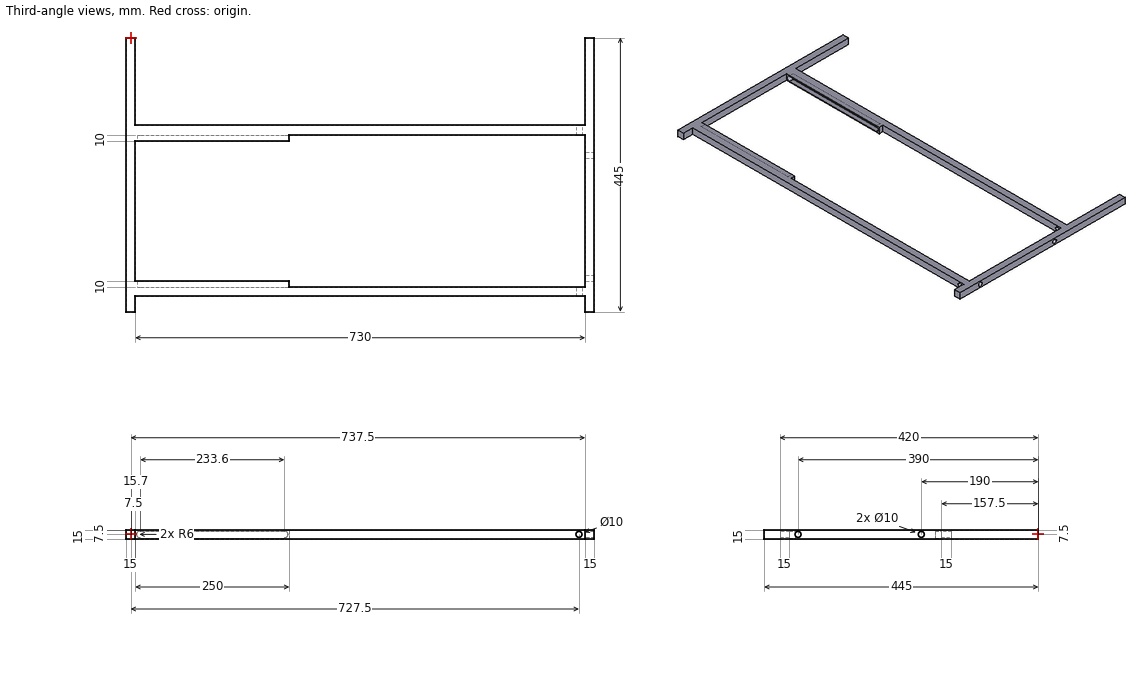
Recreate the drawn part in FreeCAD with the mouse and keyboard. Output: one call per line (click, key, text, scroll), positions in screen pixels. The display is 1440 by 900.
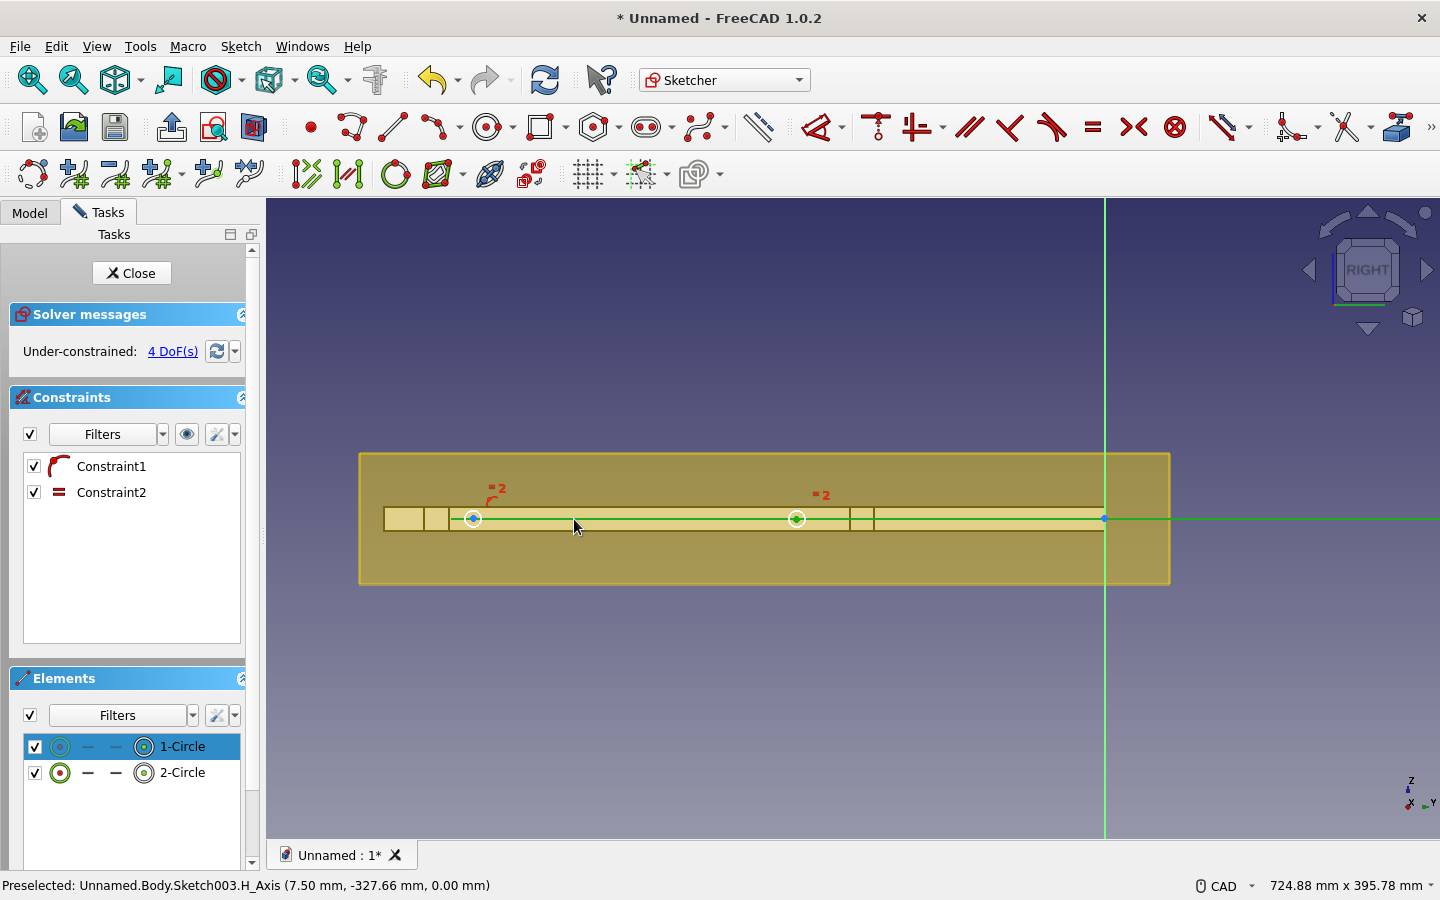
click(876, 128)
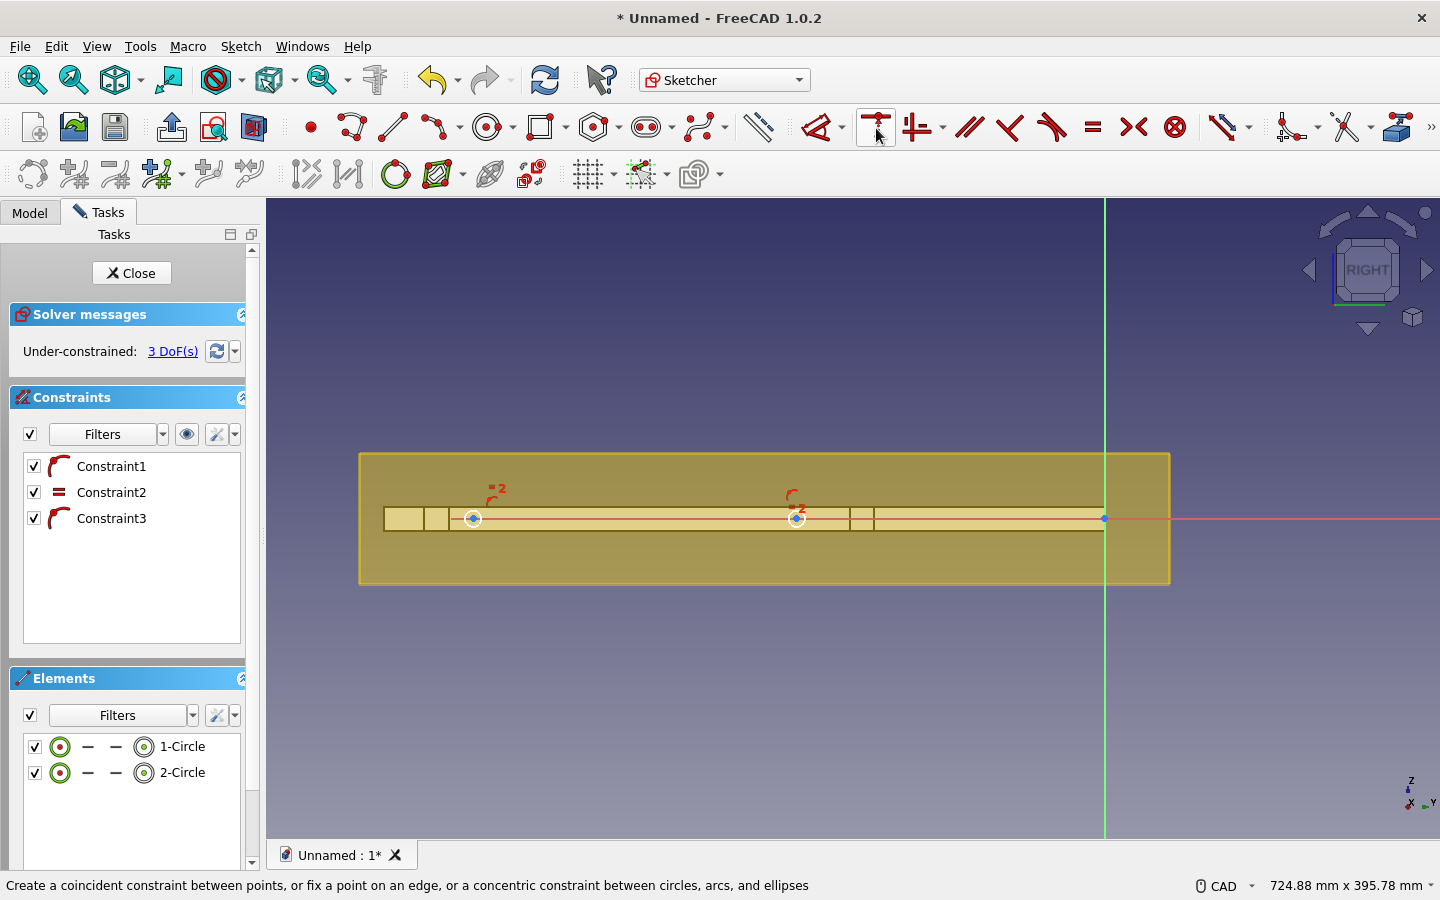
click(816, 128)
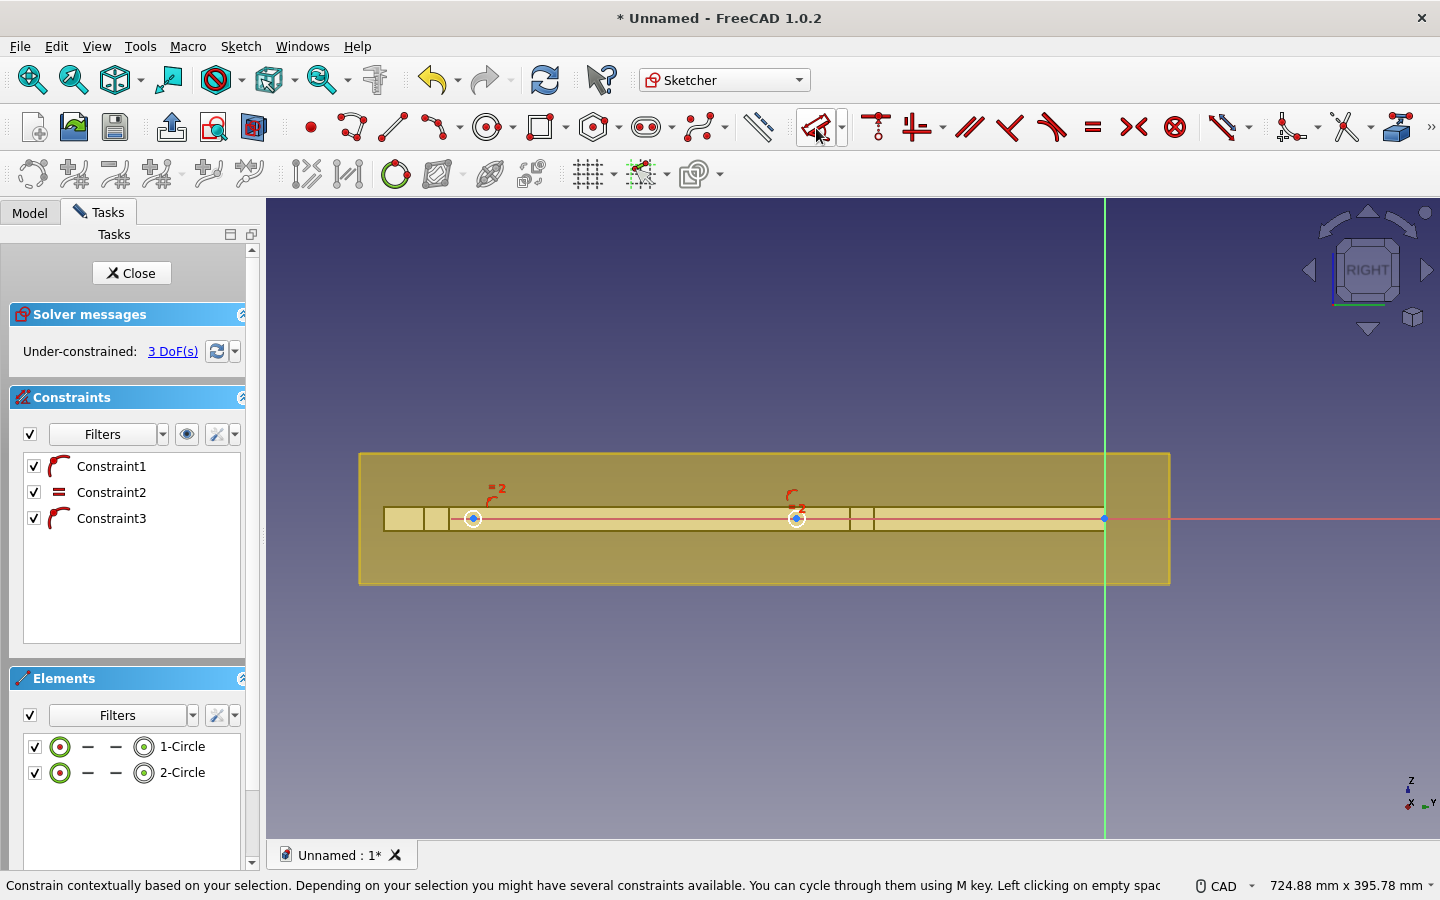
scroll(789, 519, up, 5)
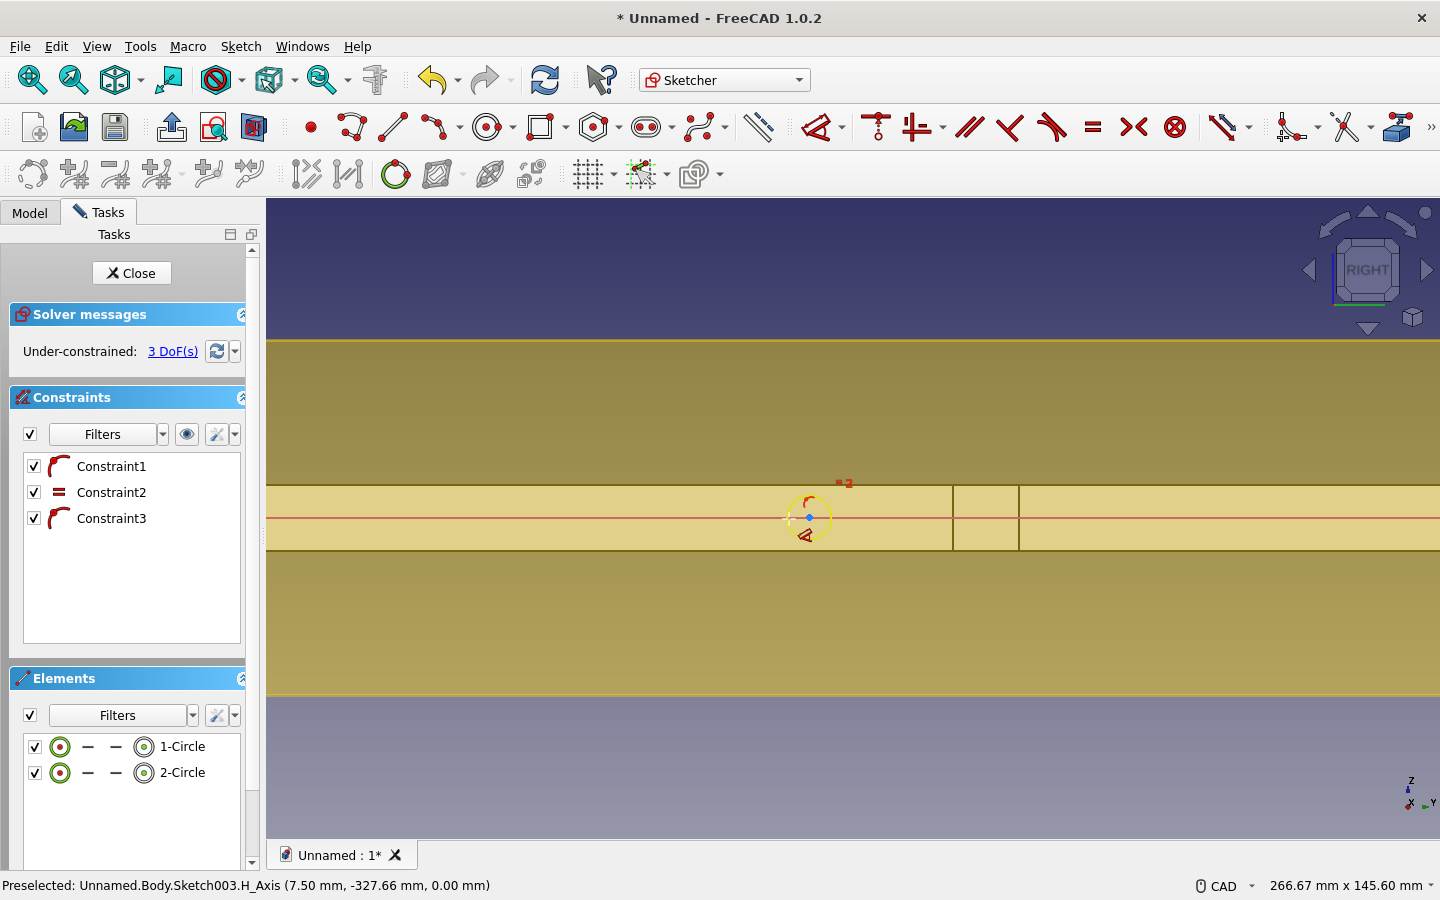
click(787, 517)
click(762, 490)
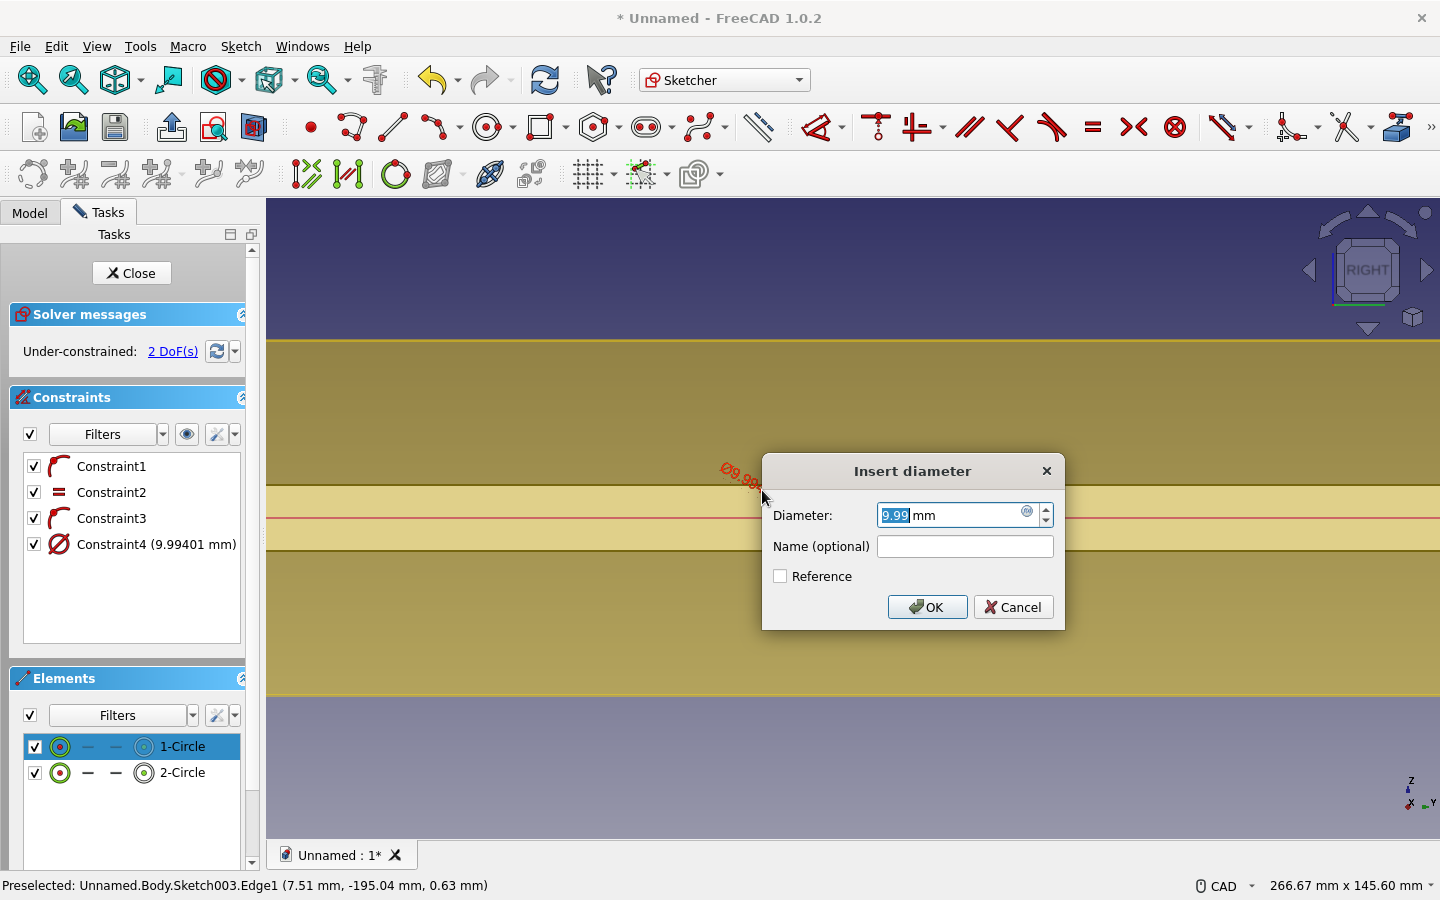
text(10)
key(Return)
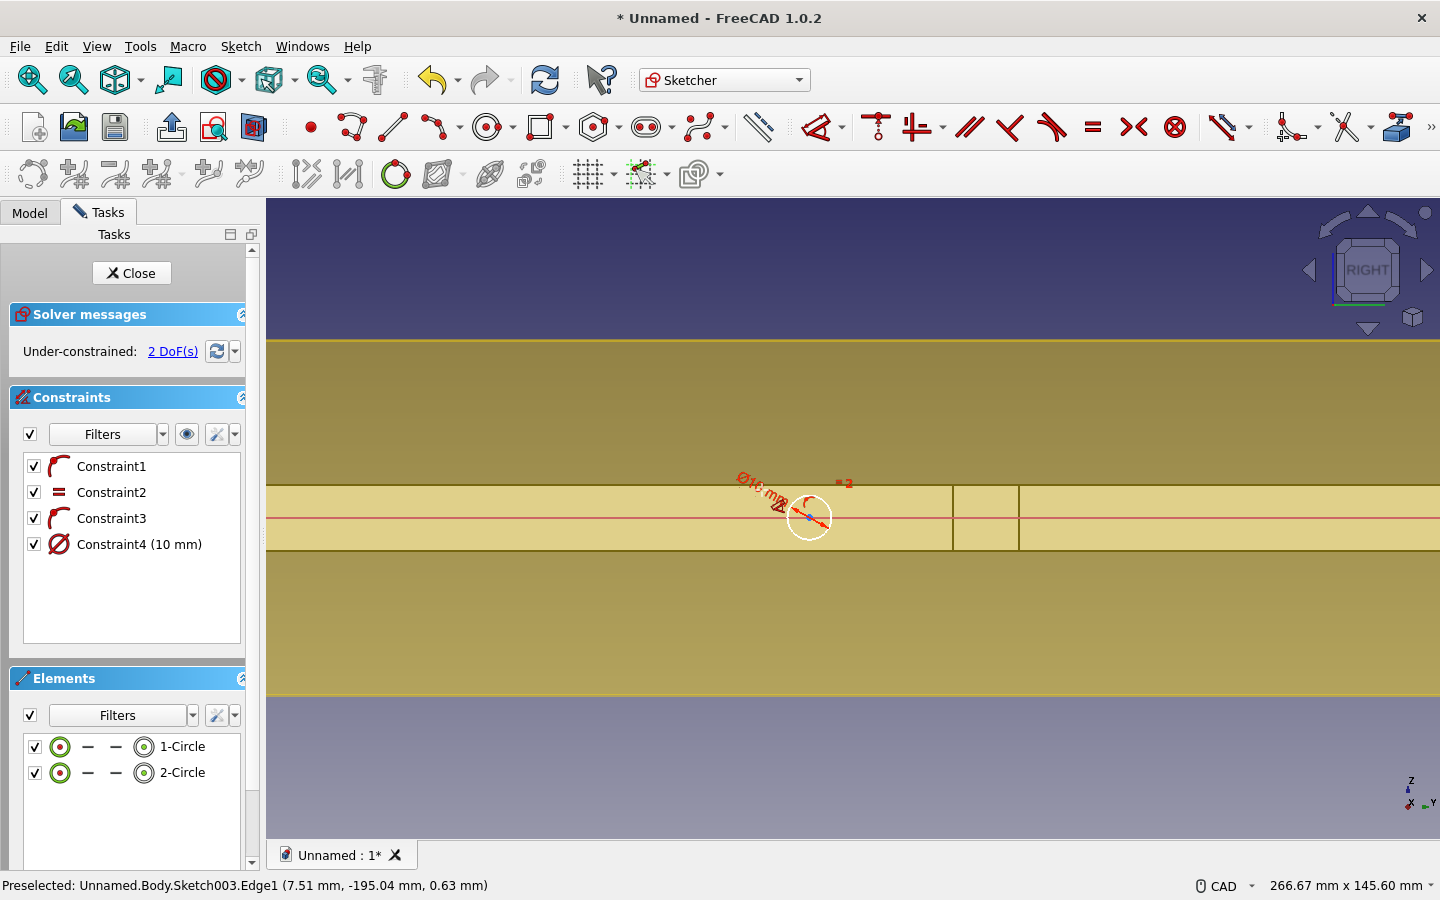
click(809, 518)
click(1042, 552)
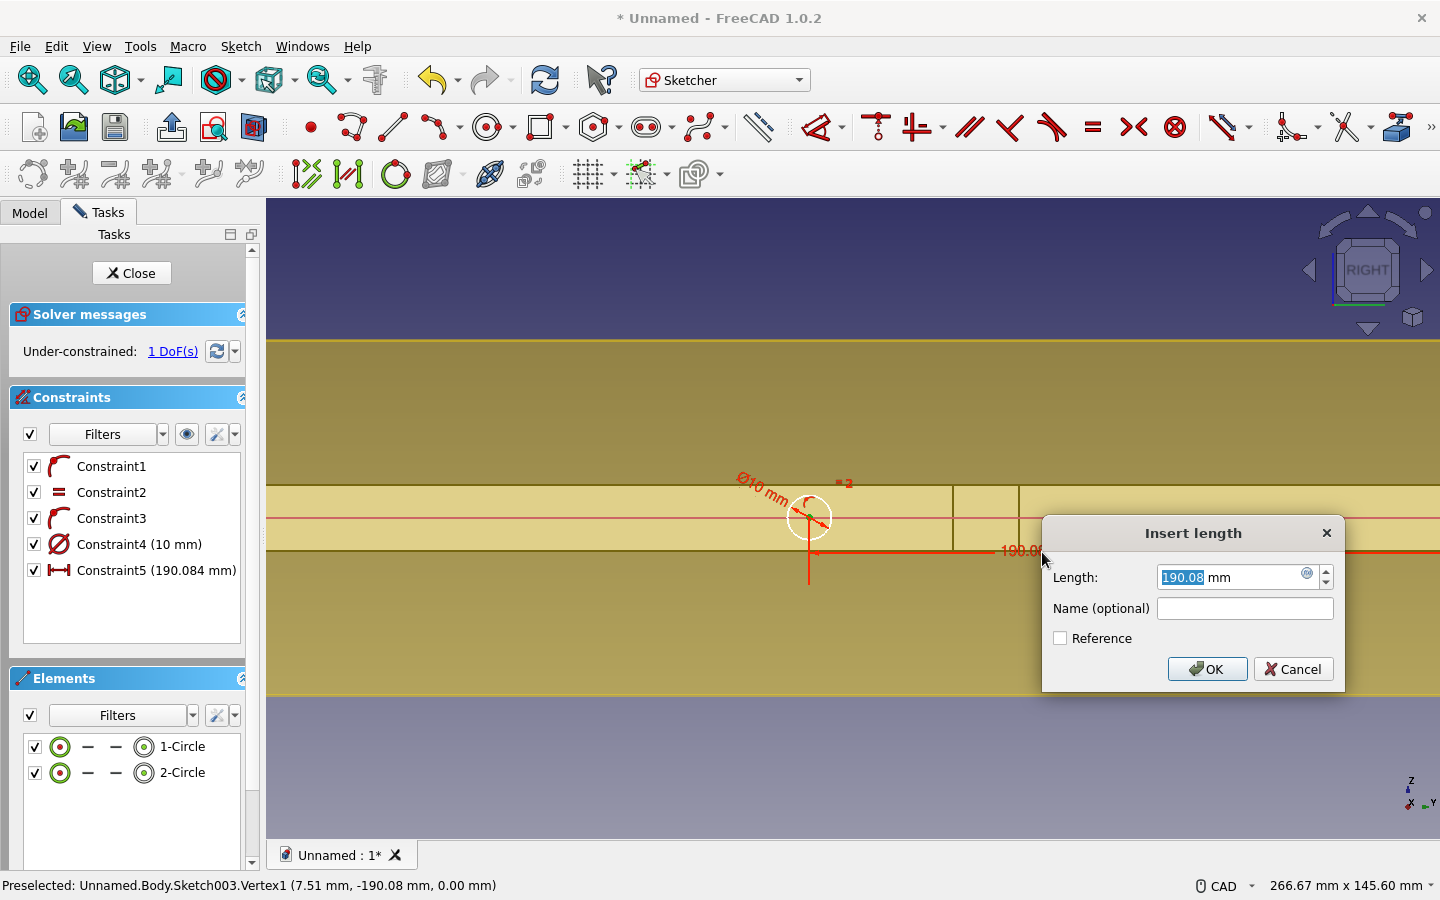
text(190)
key(Return)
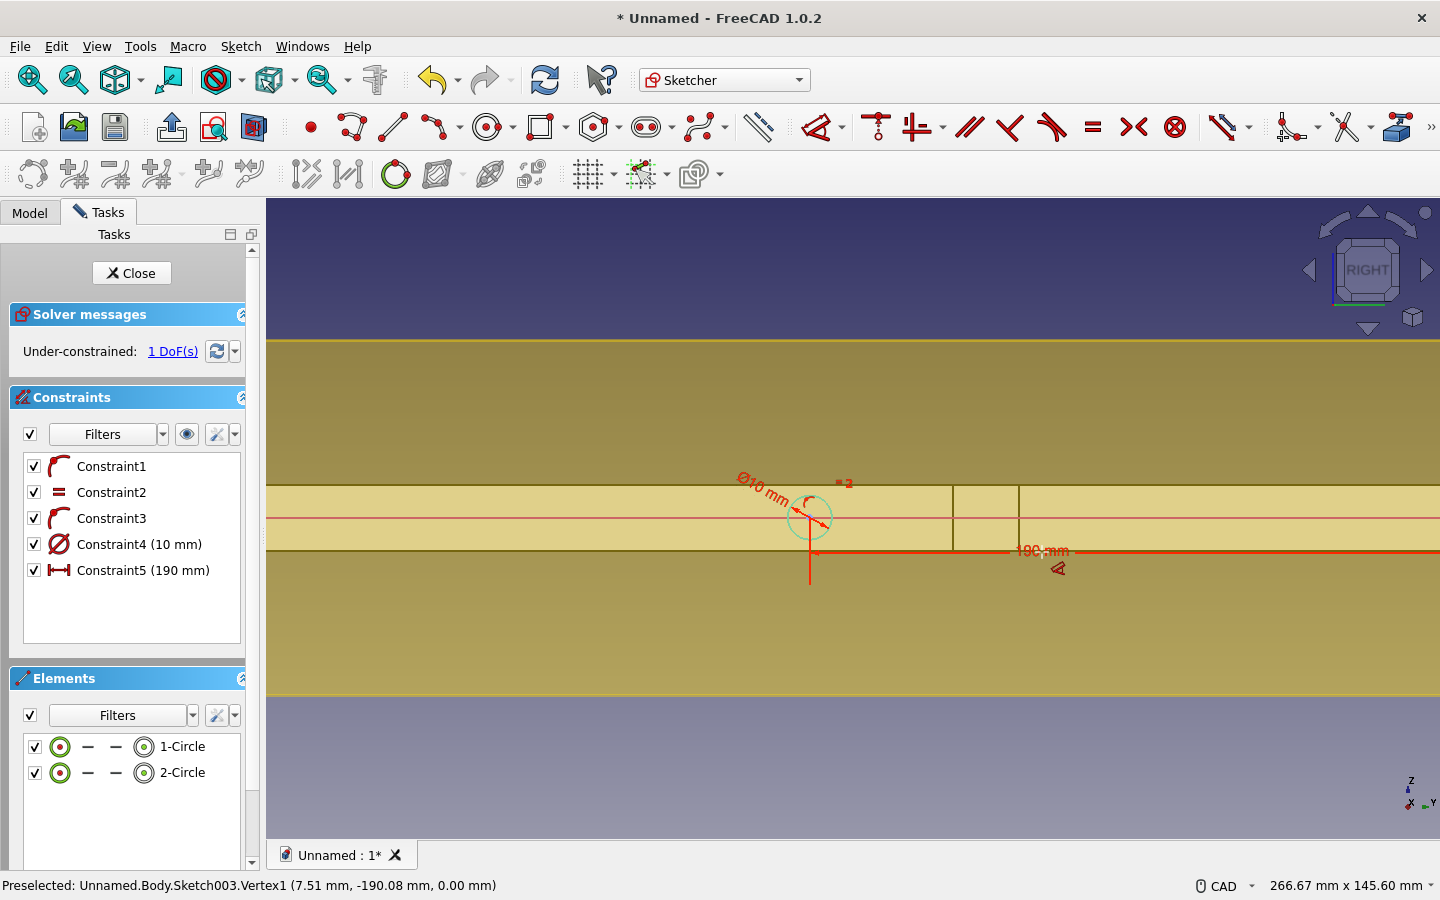
scroll(789, 519, down, 5)